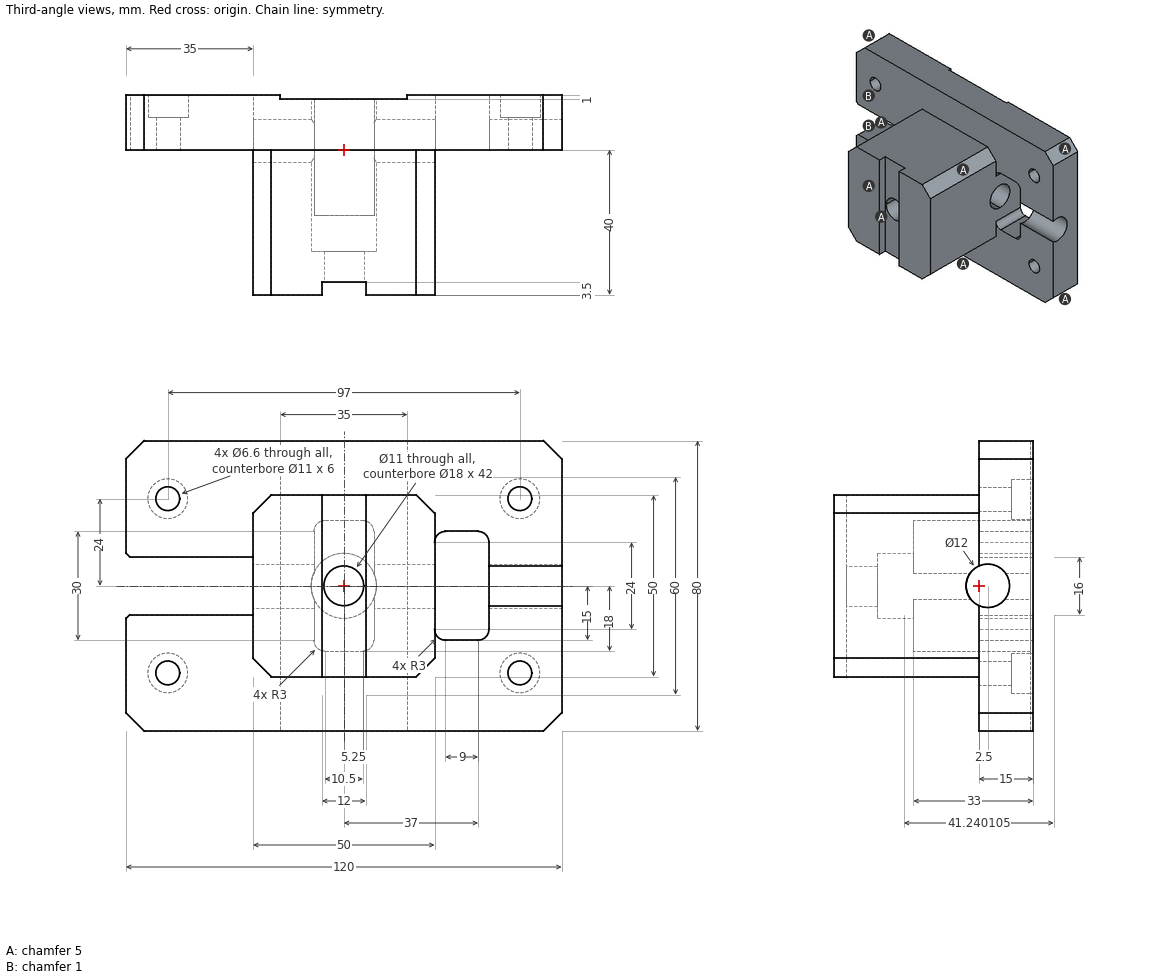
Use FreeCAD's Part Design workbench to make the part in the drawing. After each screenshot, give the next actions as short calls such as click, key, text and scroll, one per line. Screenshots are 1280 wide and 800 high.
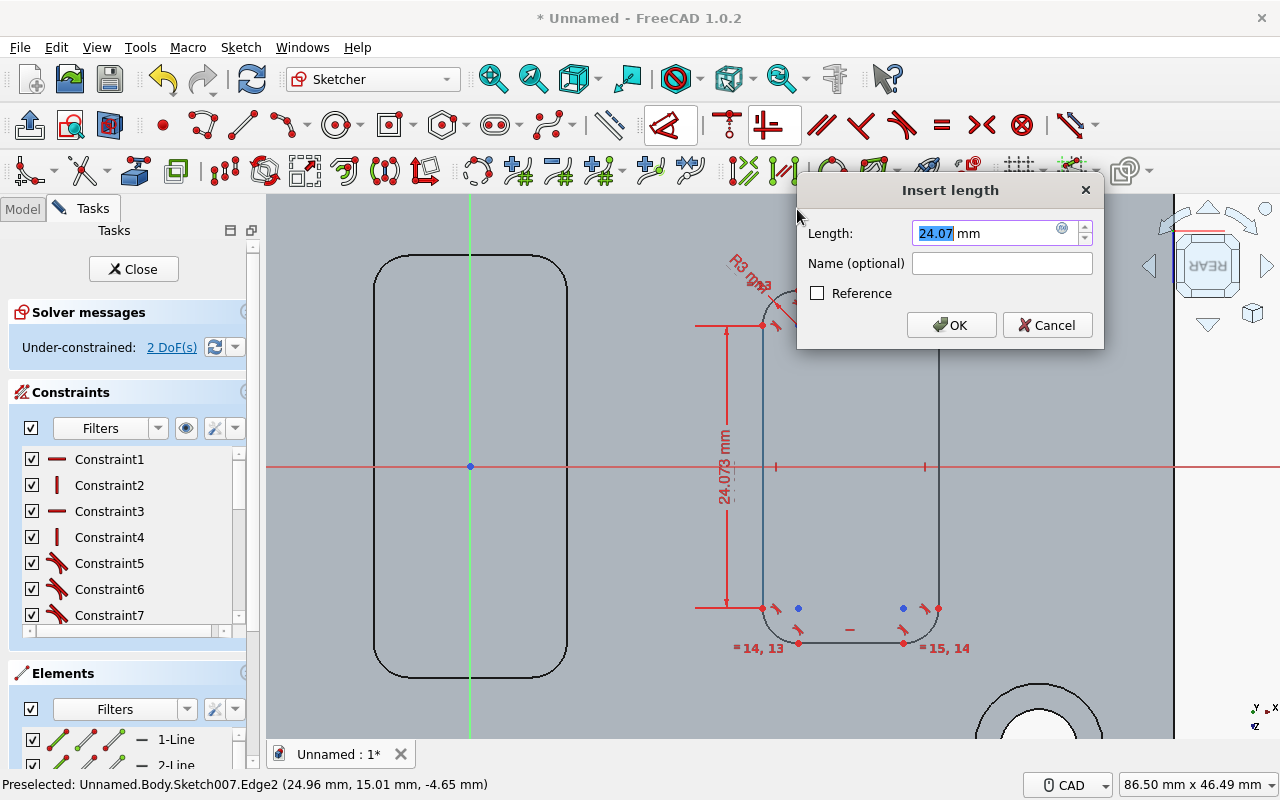
text(24)
key(Return)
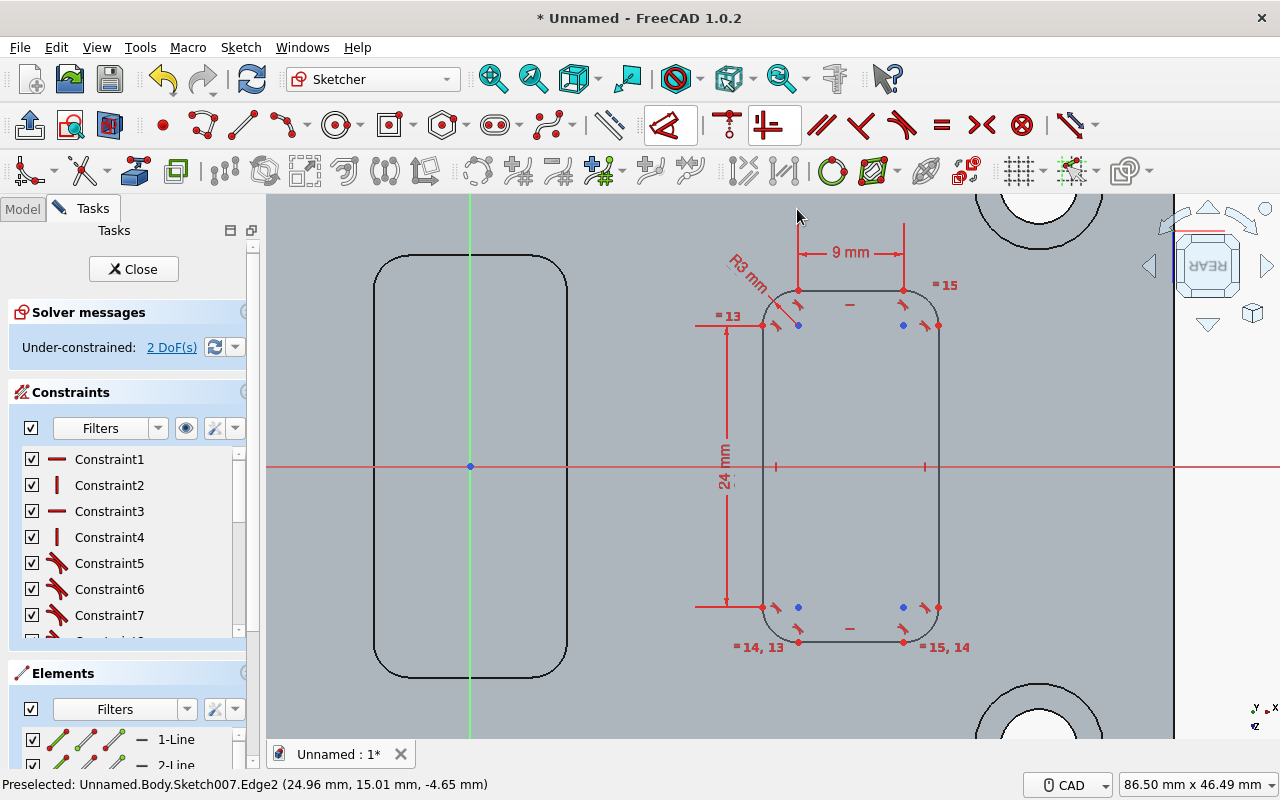
click(904, 291)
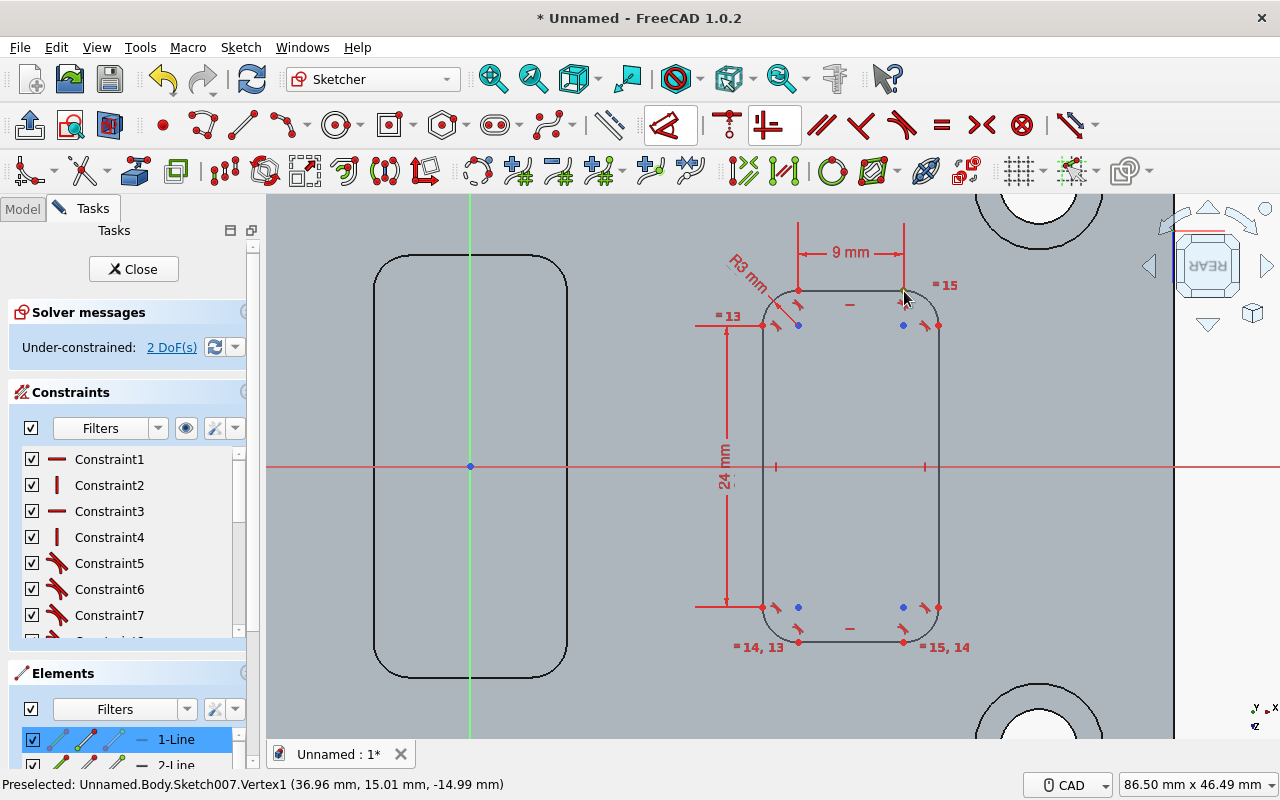
key(l)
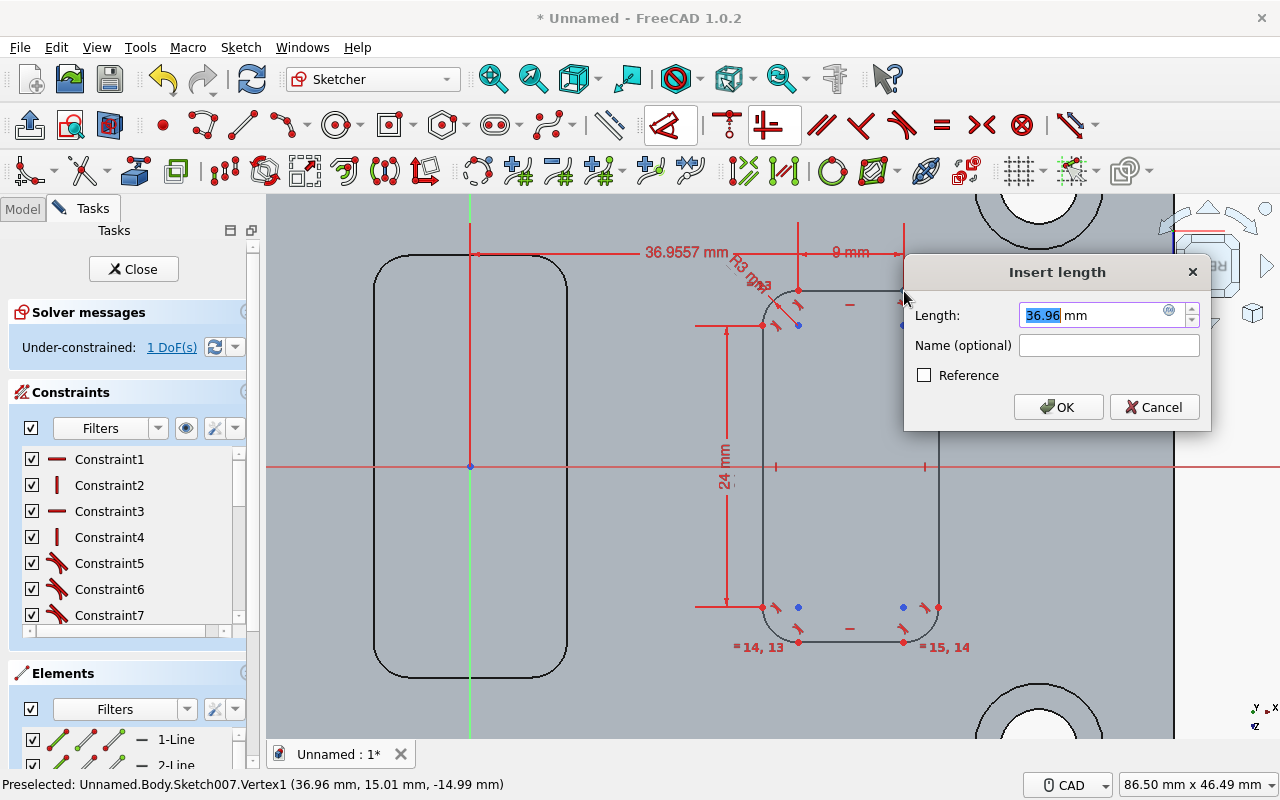
text(37)
key(Return)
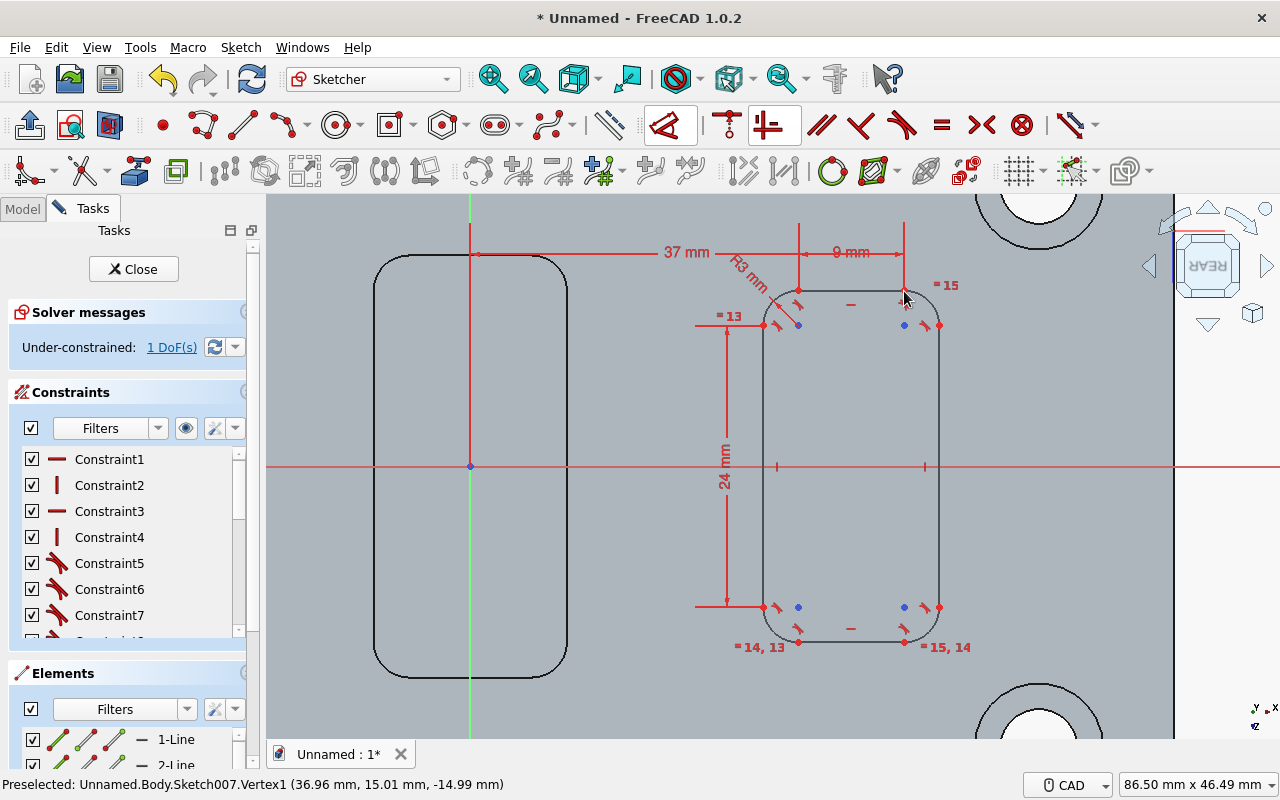
click(904, 291)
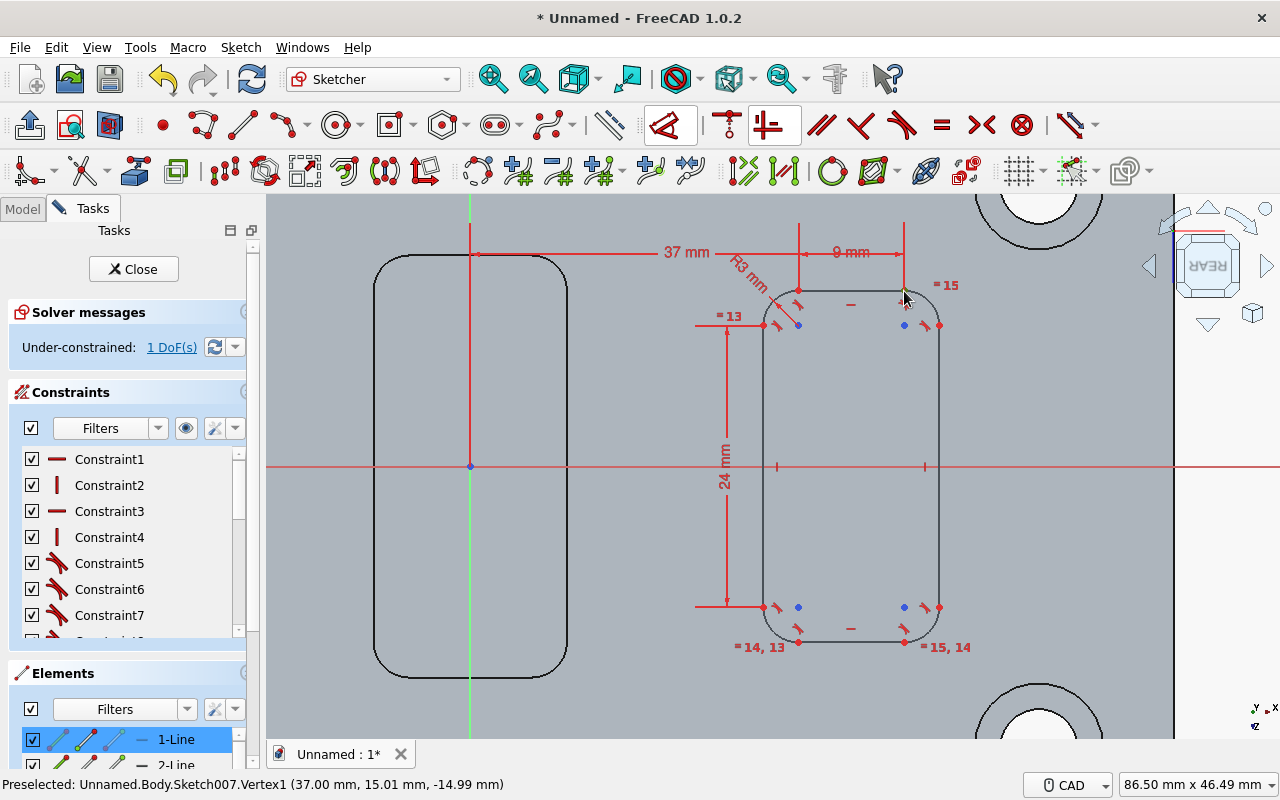
click(692, 126)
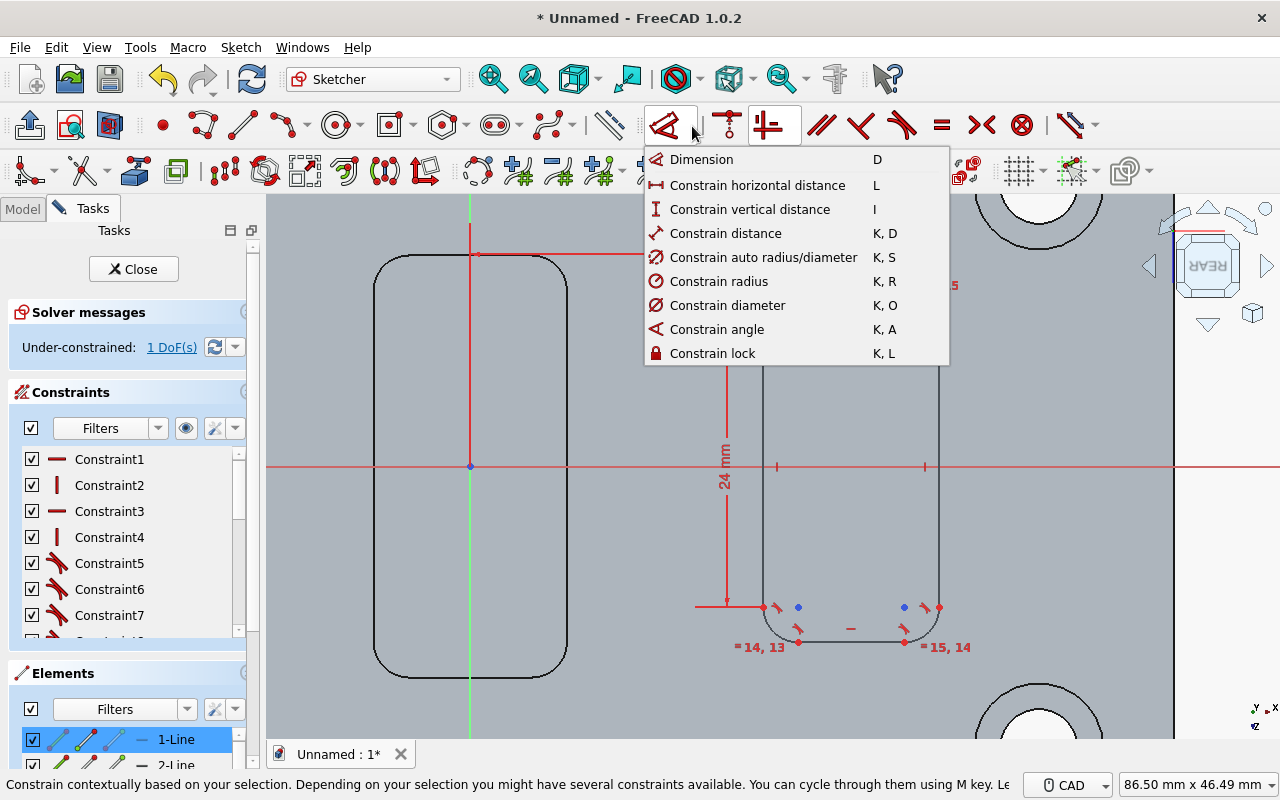
click(797, 209)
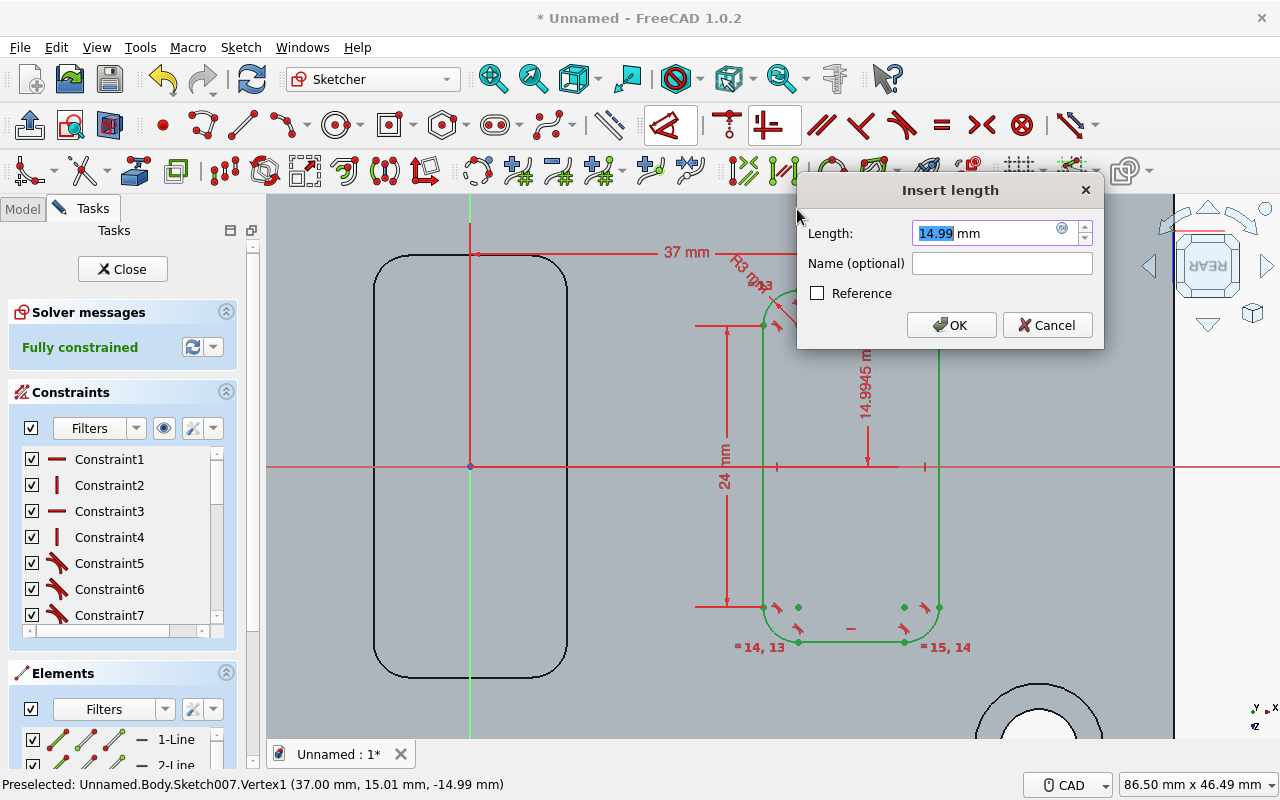
text(15)
key(Return)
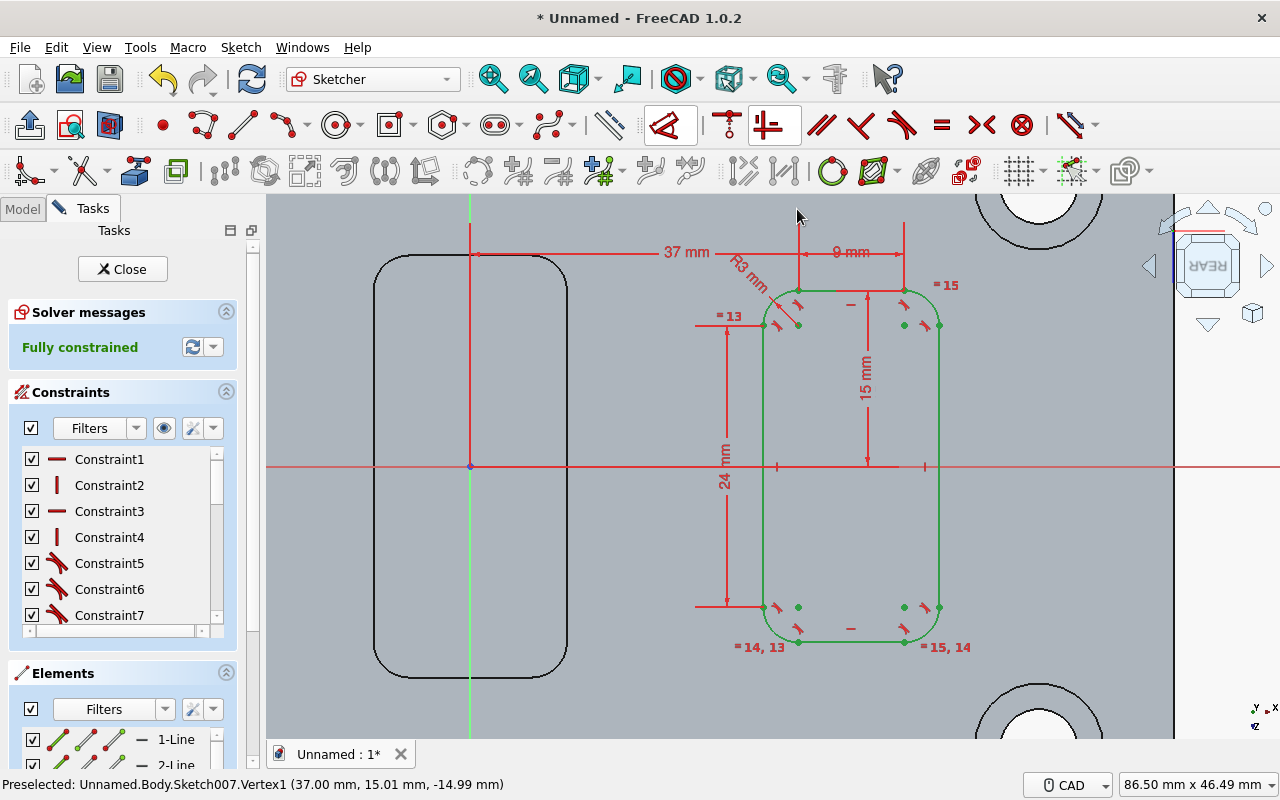
click(123, 269)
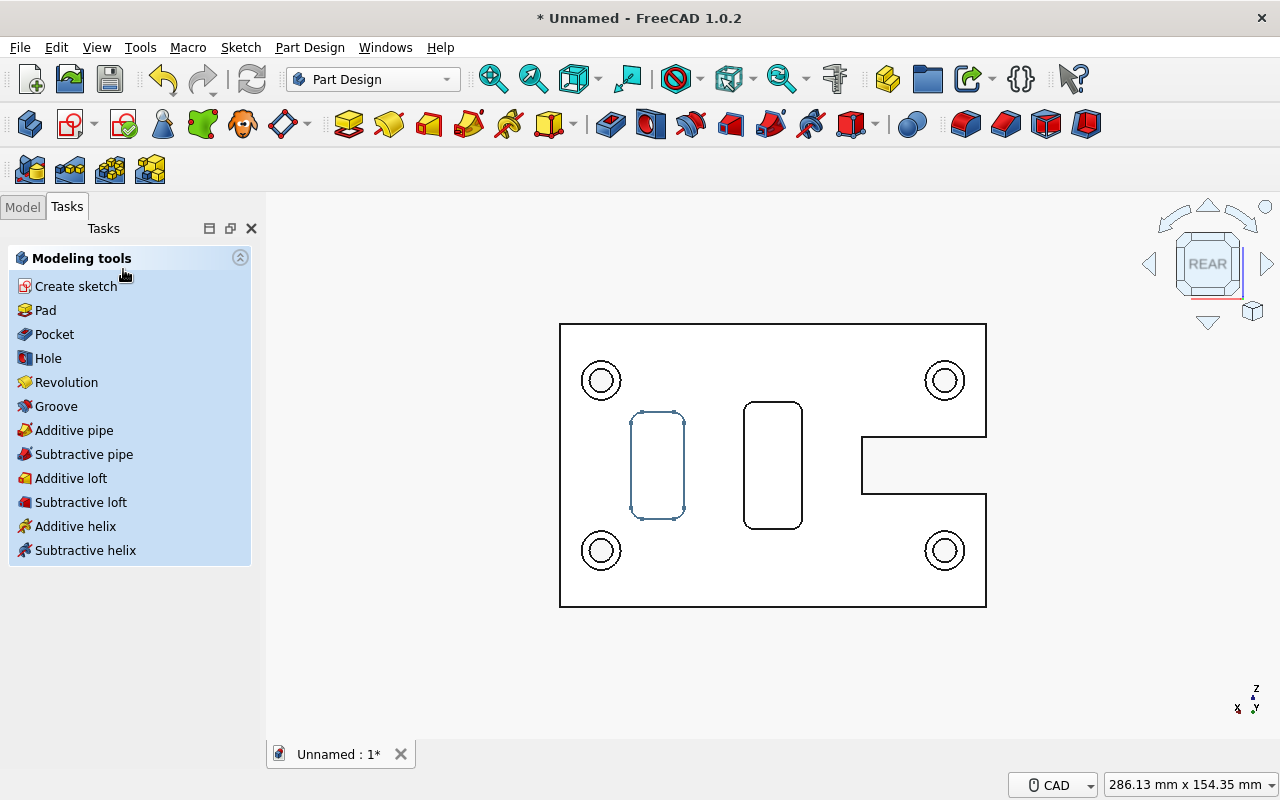
click(612, 124)